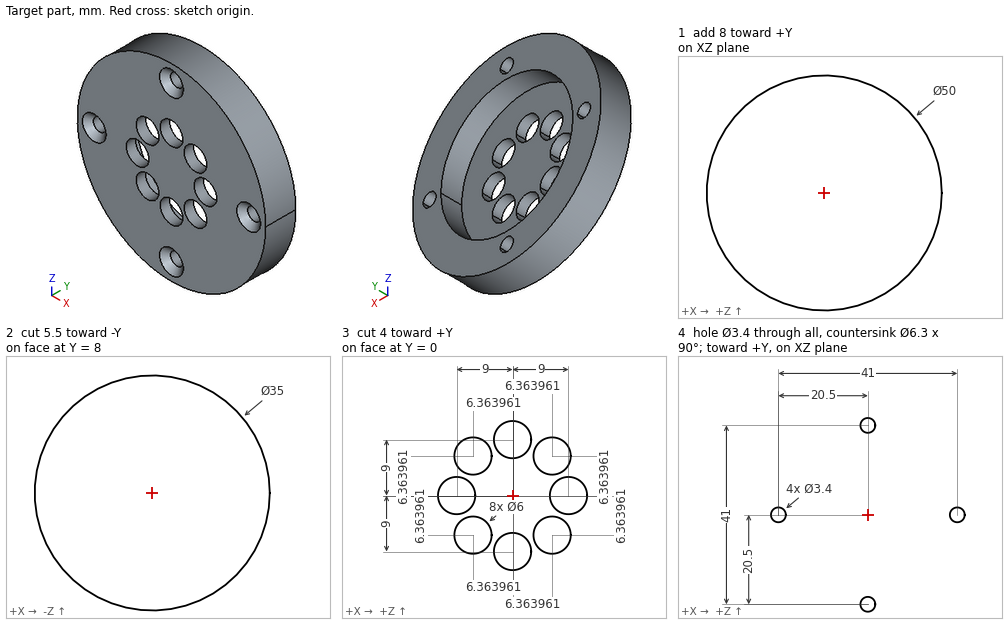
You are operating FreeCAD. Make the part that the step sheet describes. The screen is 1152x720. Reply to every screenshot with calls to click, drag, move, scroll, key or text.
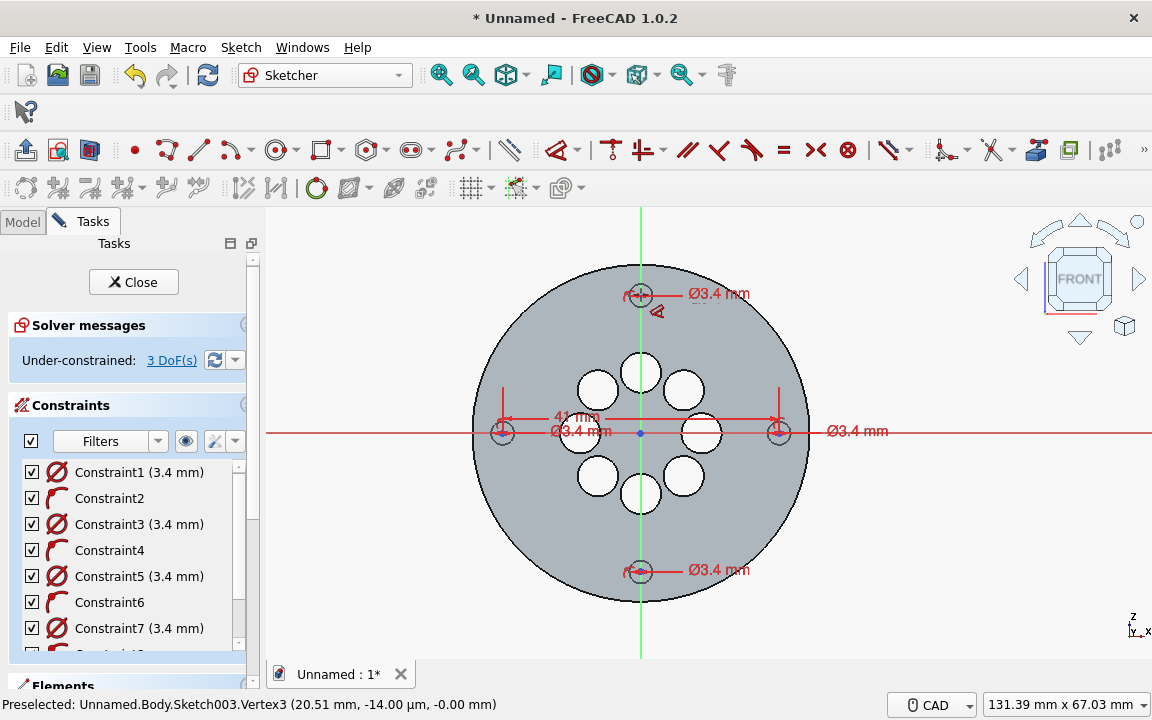
click(641, 572)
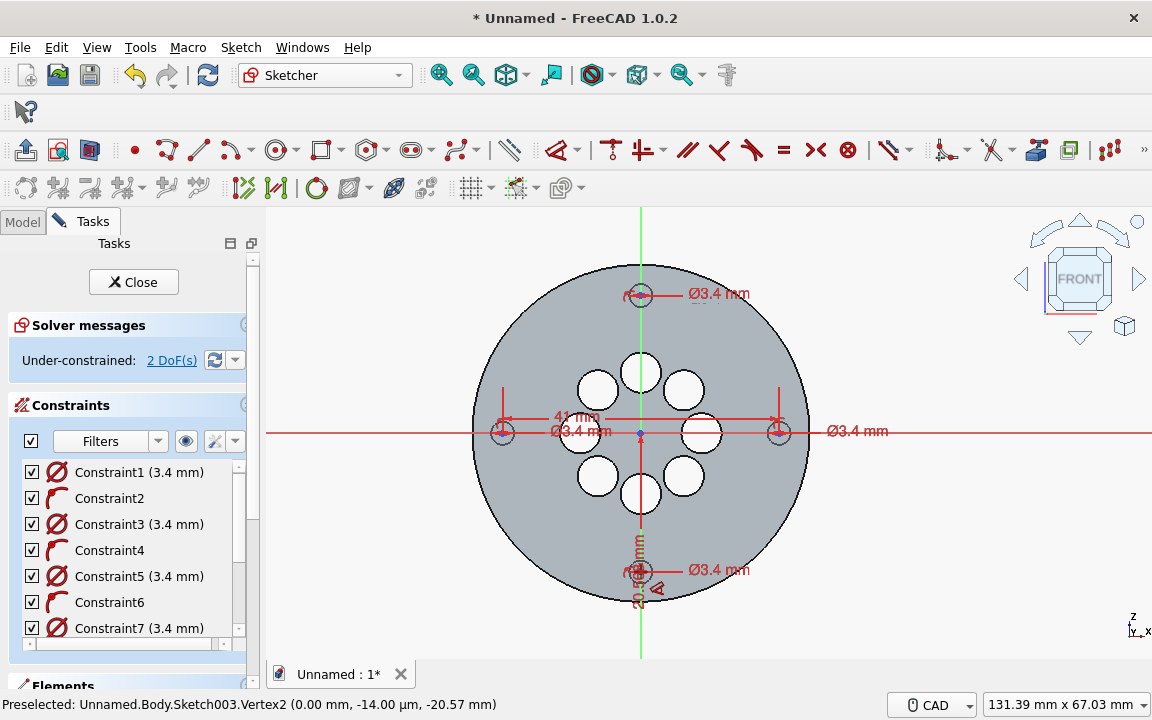
click(641, 296)
click(675, 370)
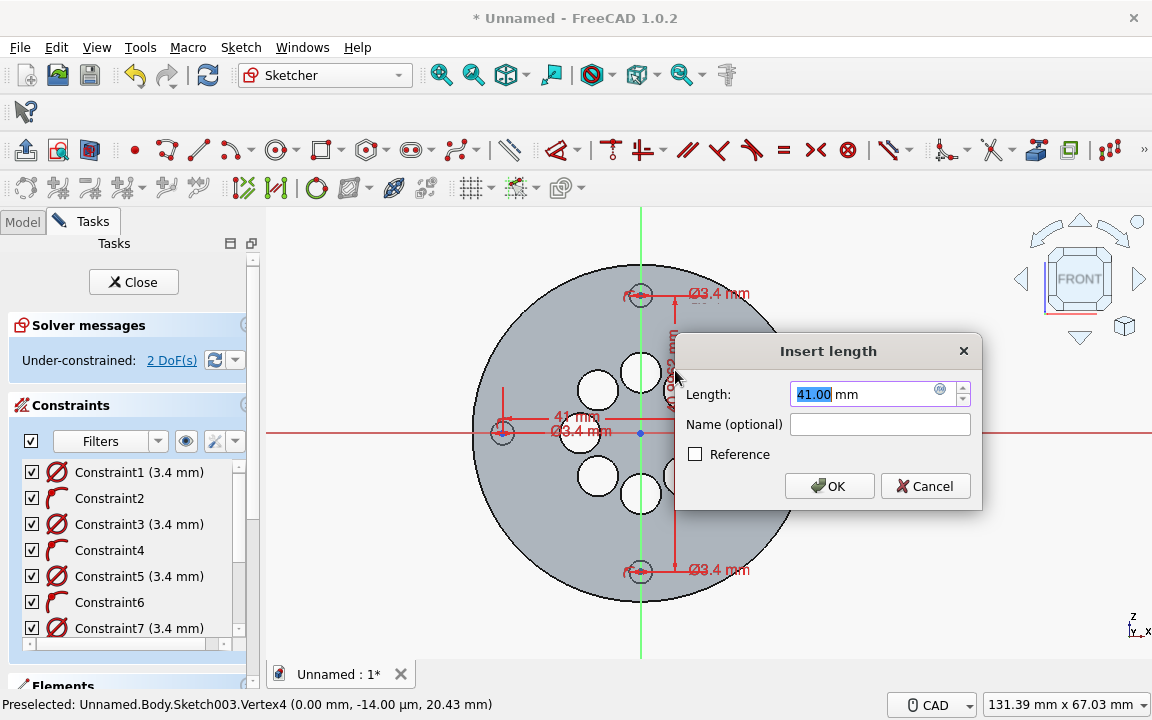
text(41)
key(Return)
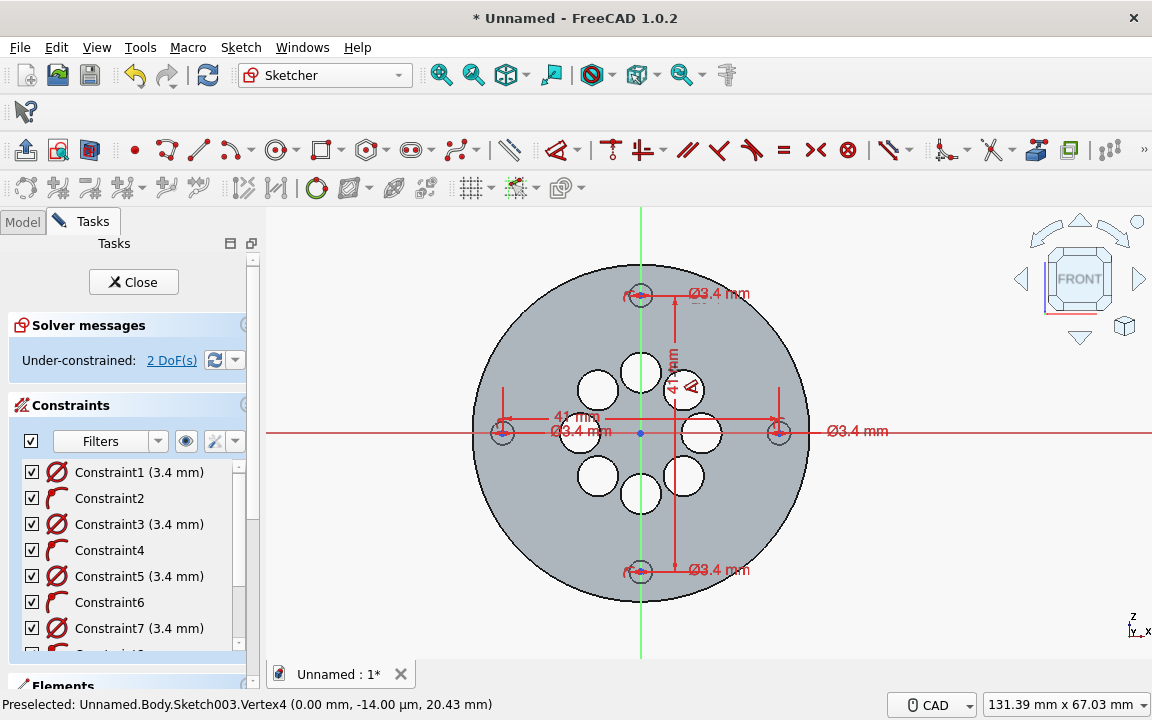
click(503, 433)
click(572, 467)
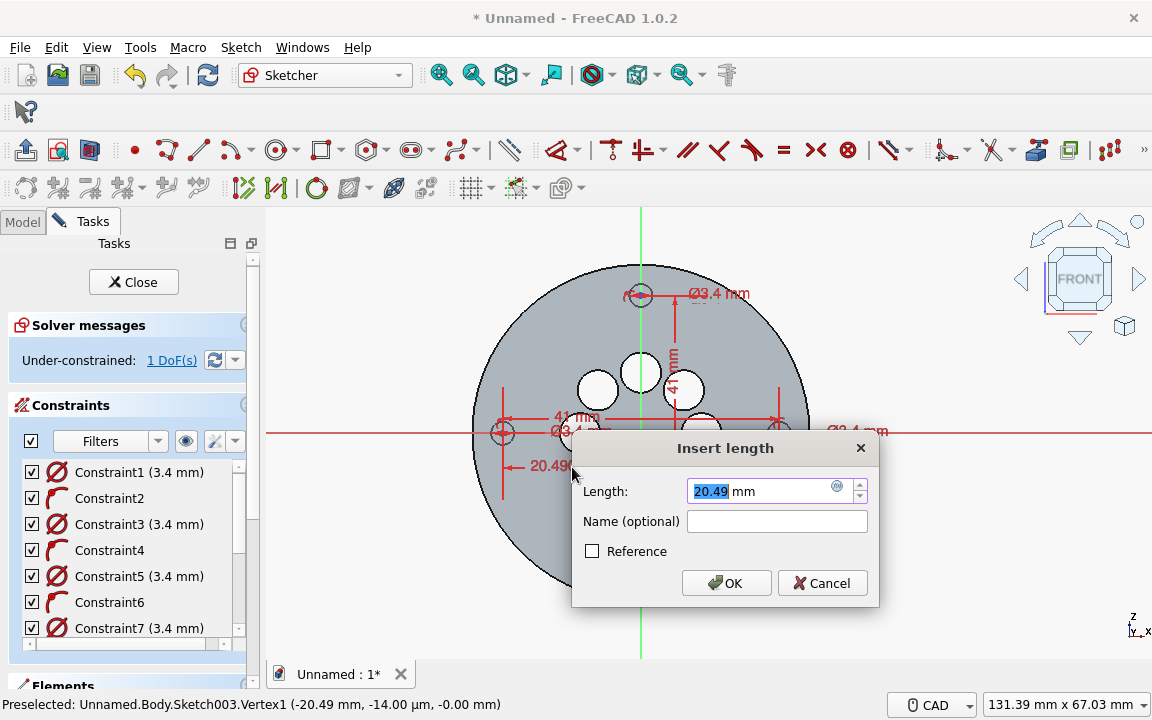
text(20.5)
key(Return)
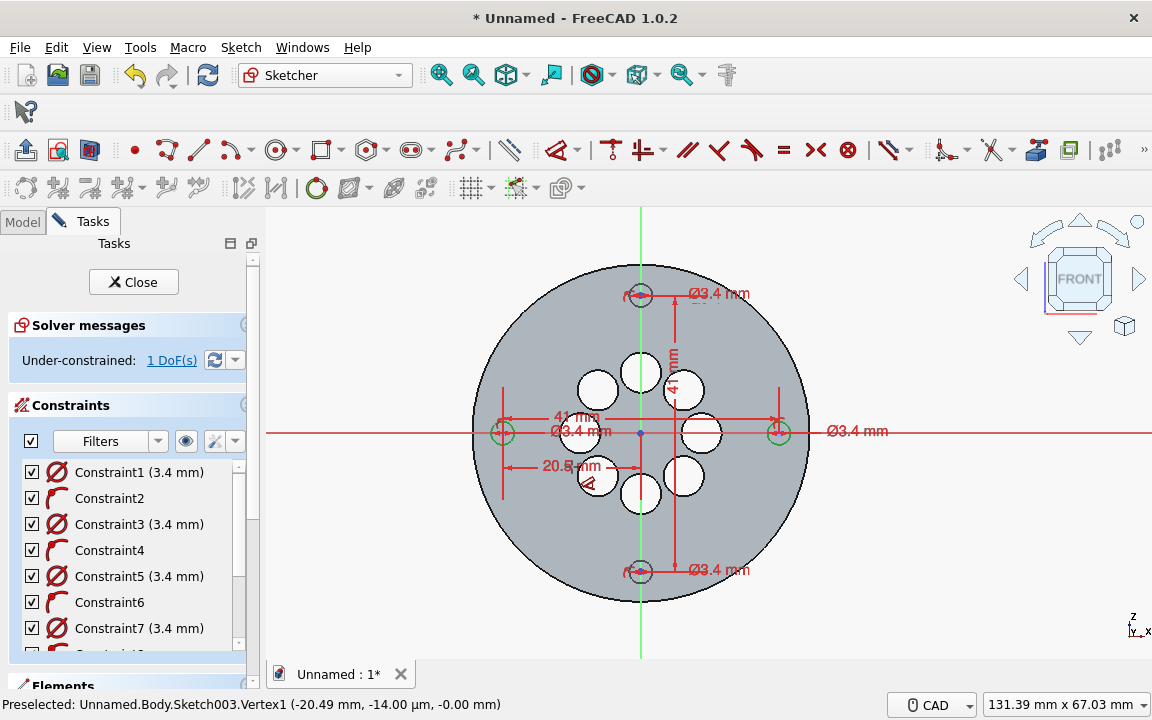
click(641, 572)
click(675, 503)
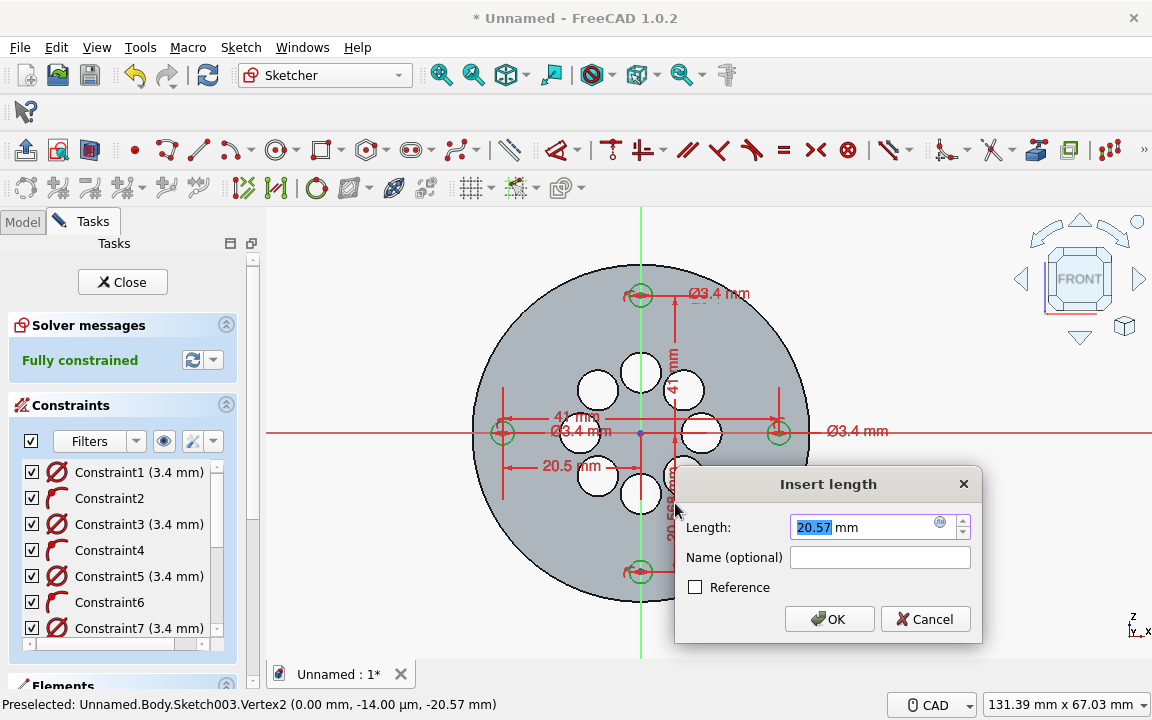
text(20.5)
key(Return)
key(Escape)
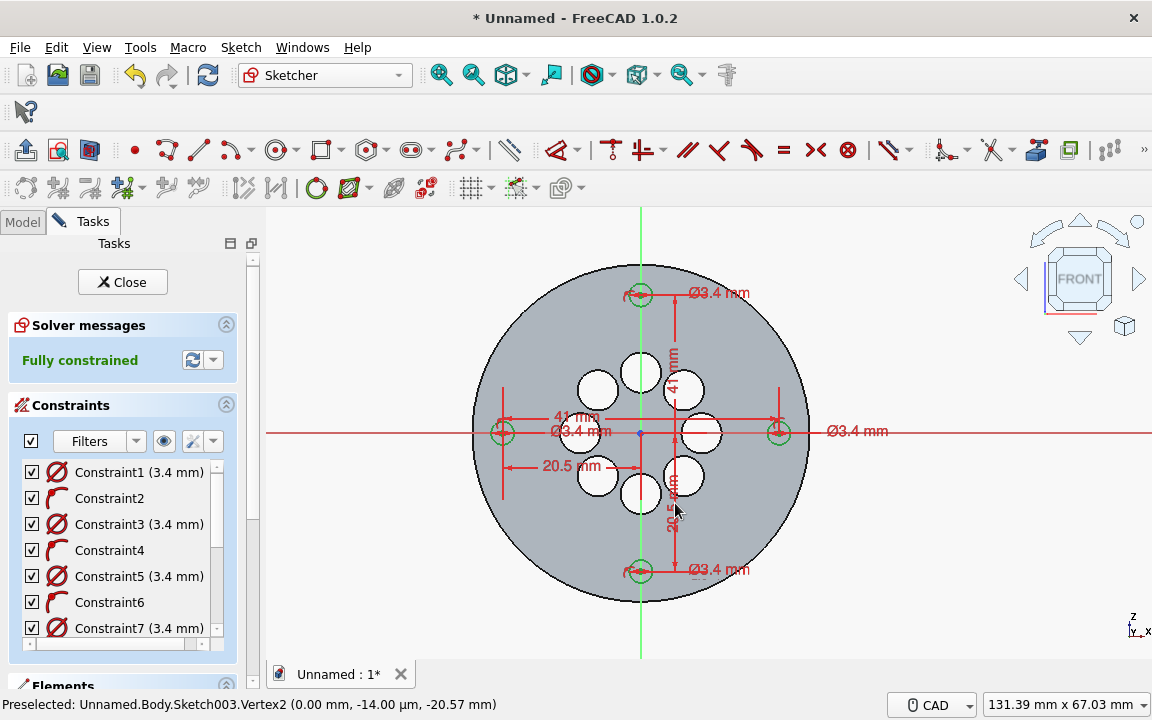
click(123, 282)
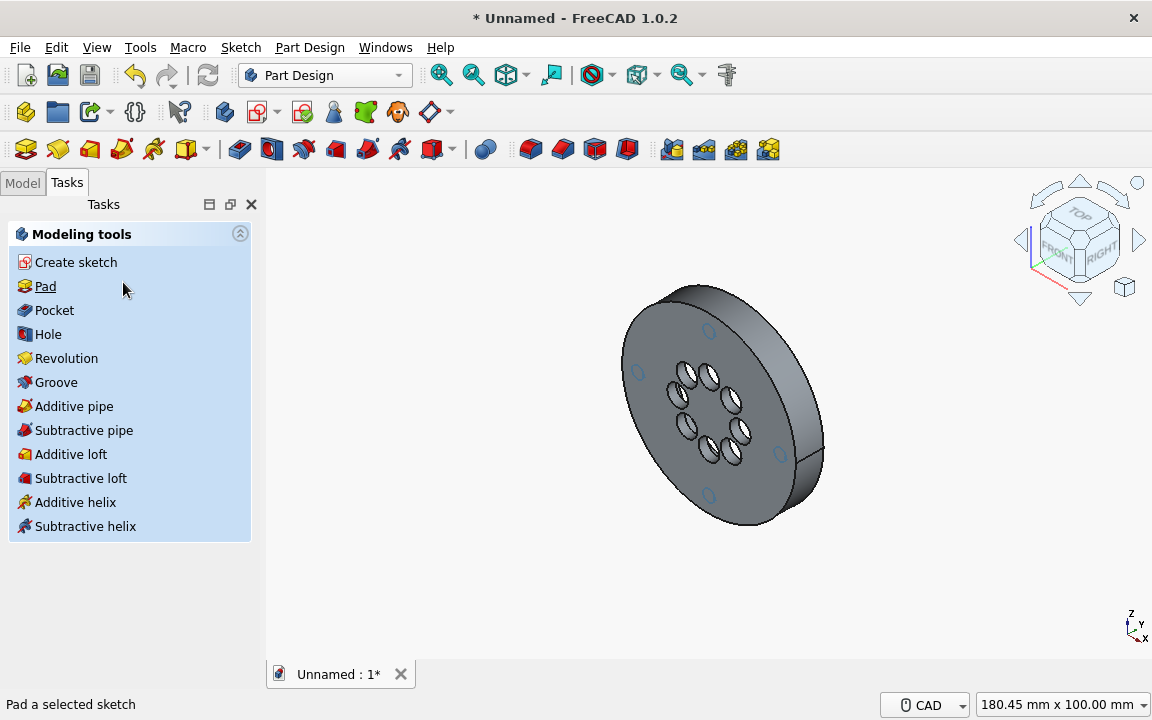
click(272, 150)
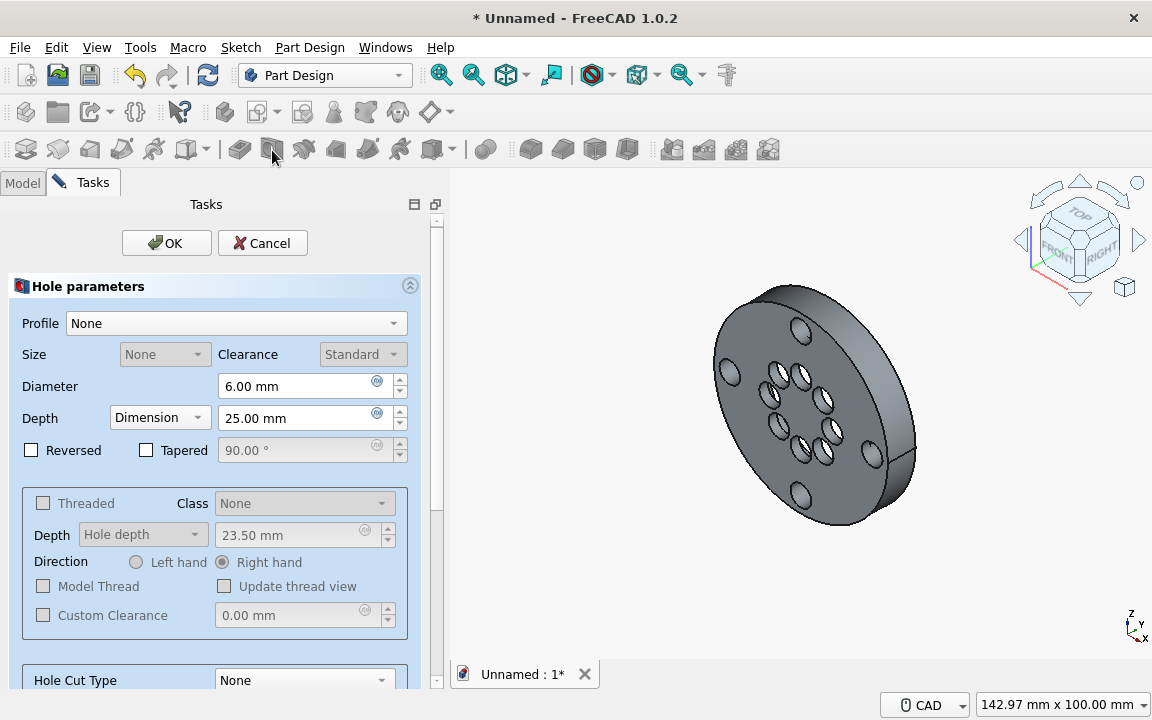
triple_click(305, 386)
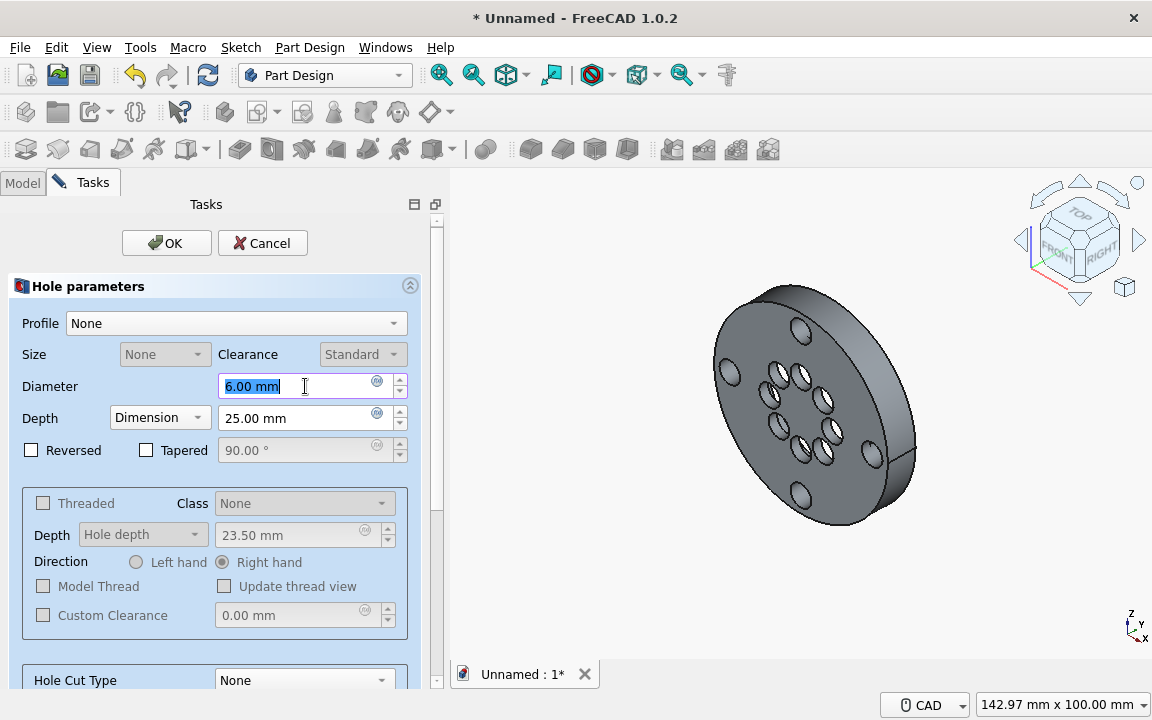
text(3.4)
key(Tab)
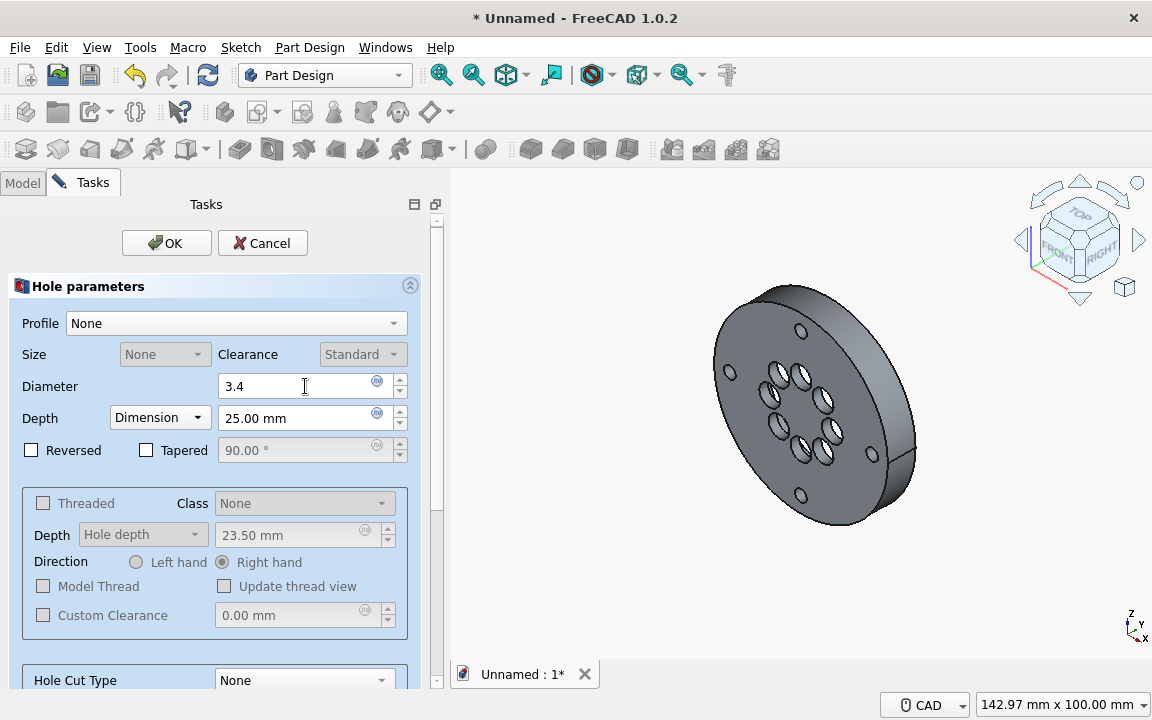
click(161, 418)